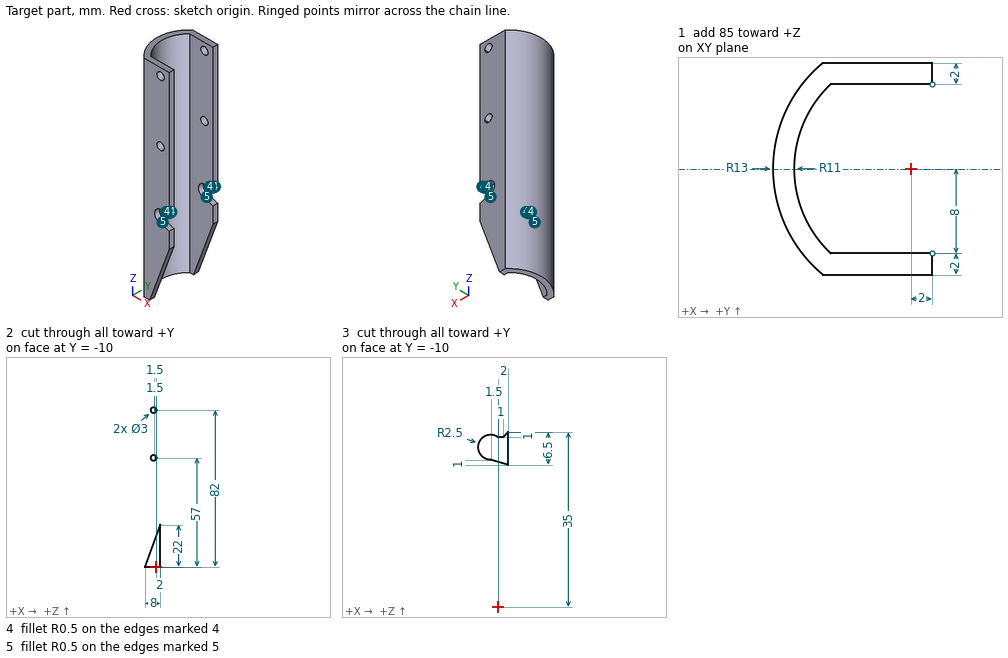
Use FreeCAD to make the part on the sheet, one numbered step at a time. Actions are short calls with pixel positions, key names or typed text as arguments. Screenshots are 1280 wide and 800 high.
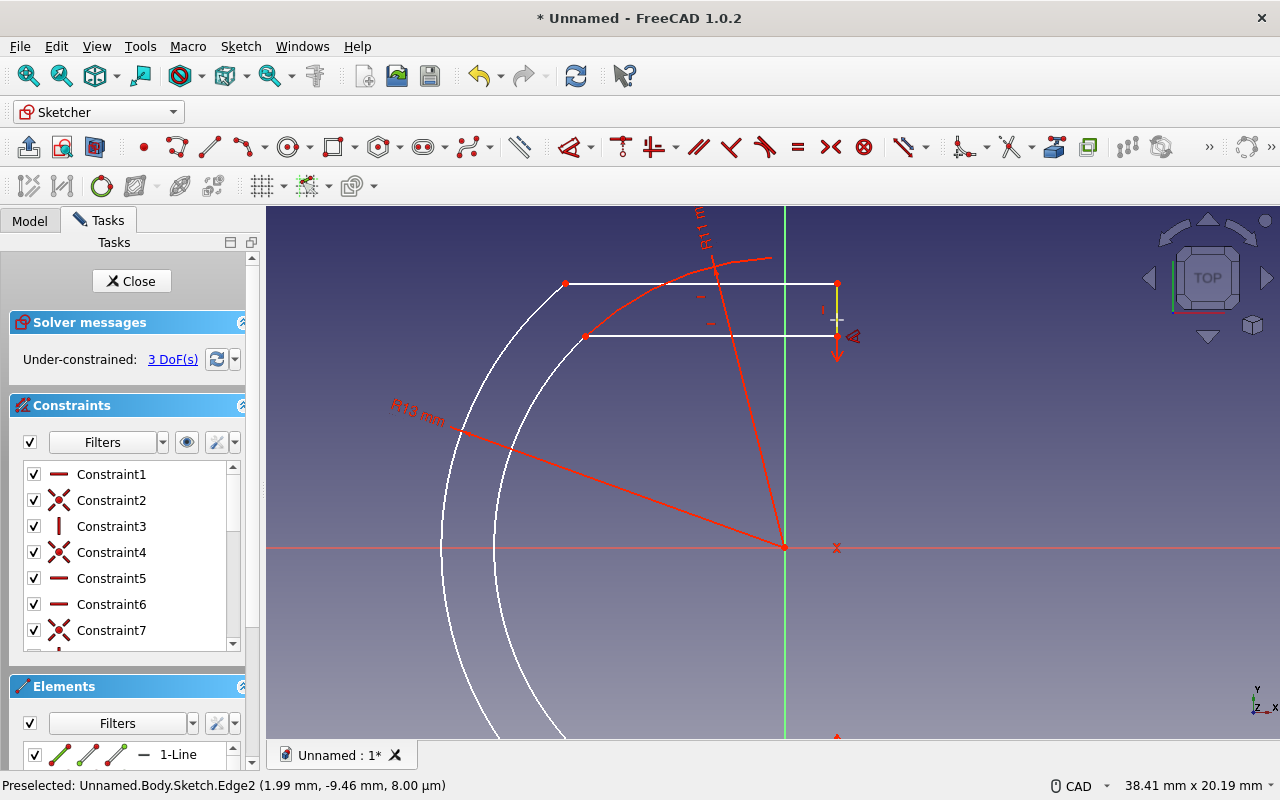
click(837, 320)
click(871, 310)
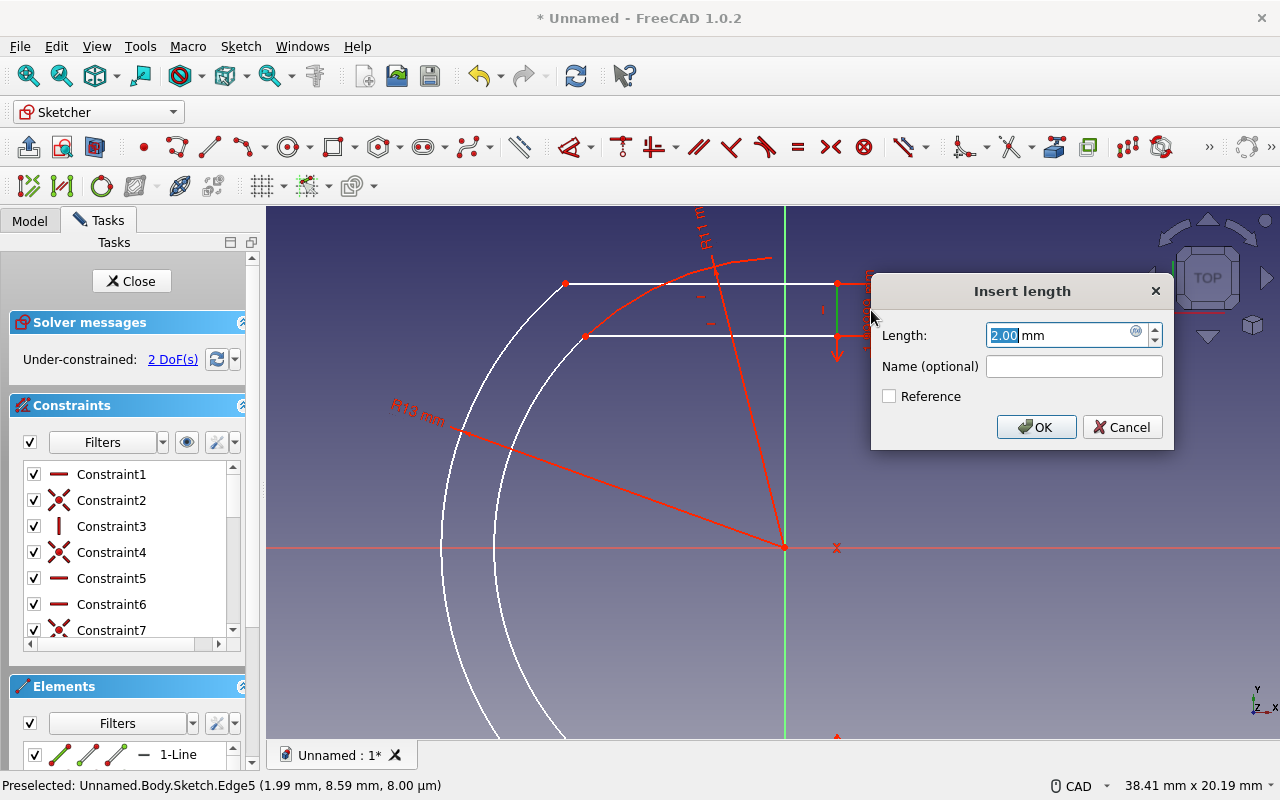
text(2)
key(Return)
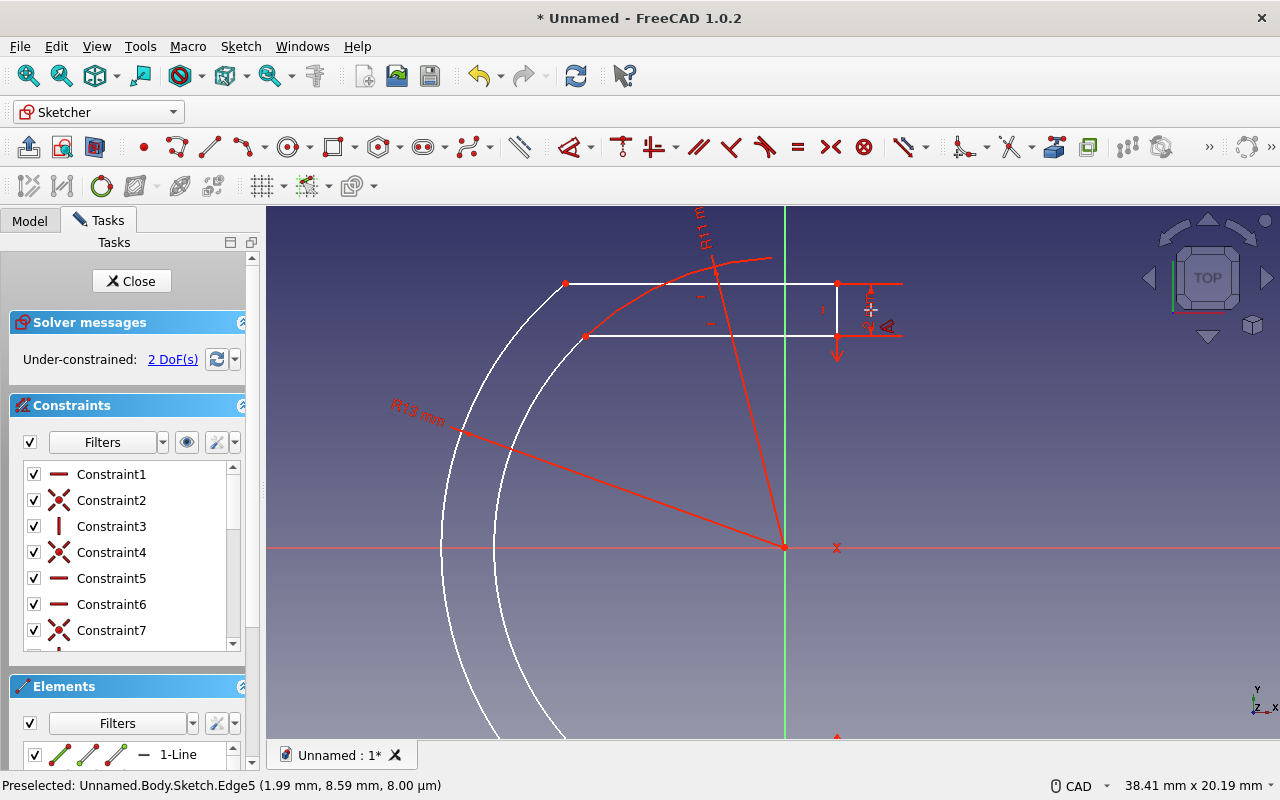
scroll(837, 319, down, 2)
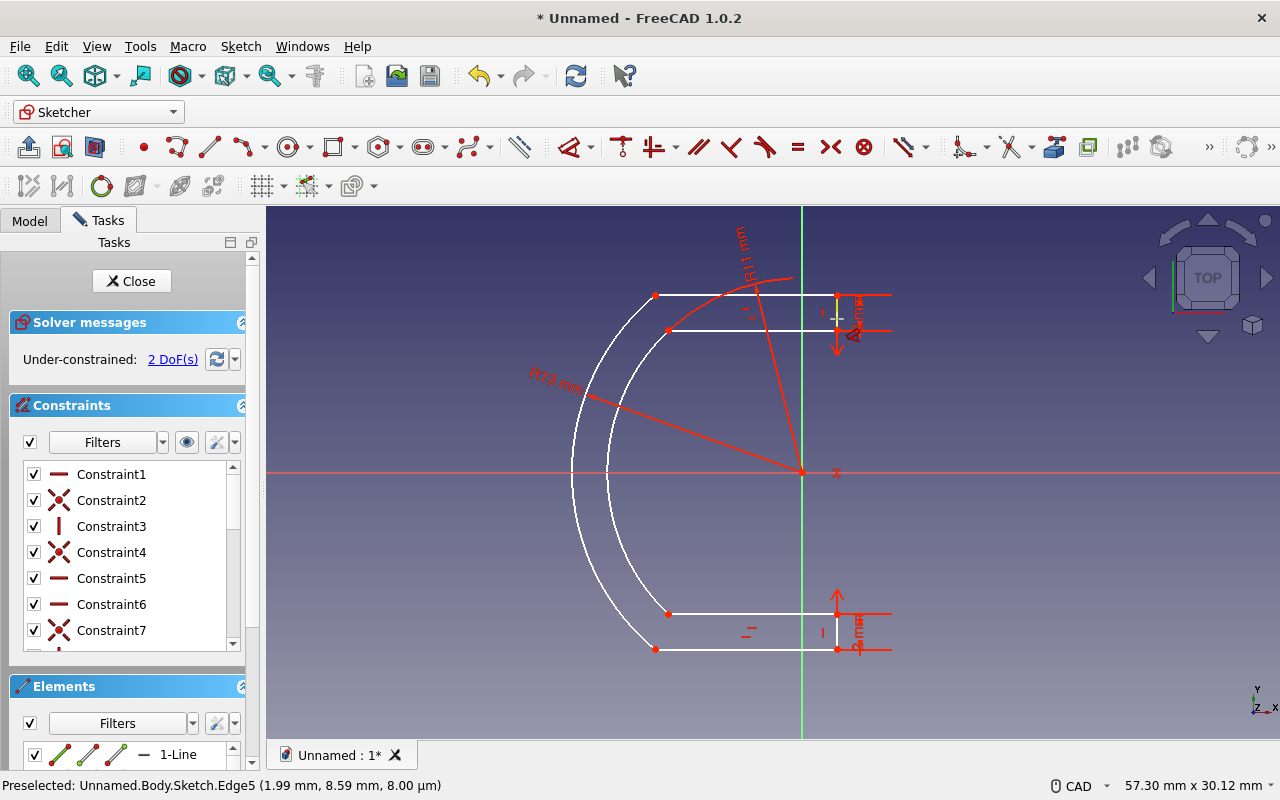
click(837, 650)
click(820, 684)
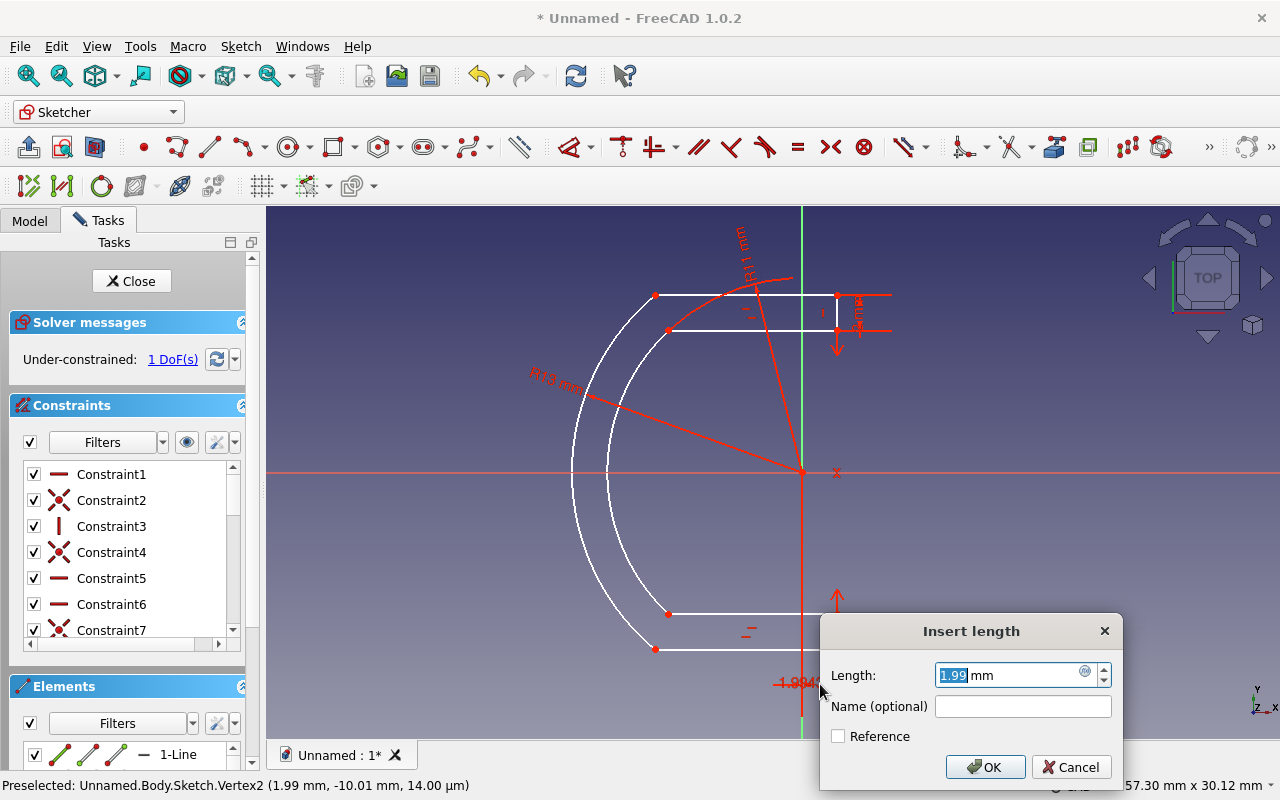
text(2)
key(Return)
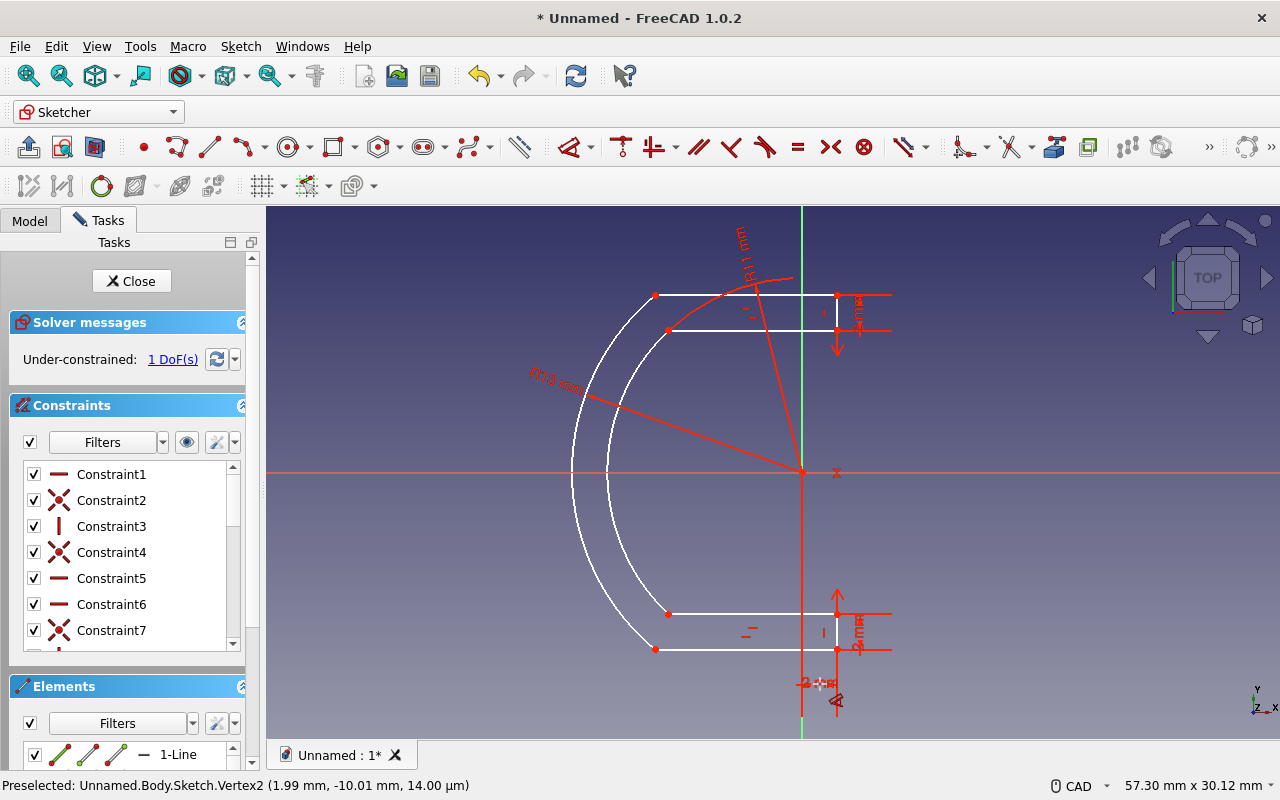
click(837, 614)
click(871, 543)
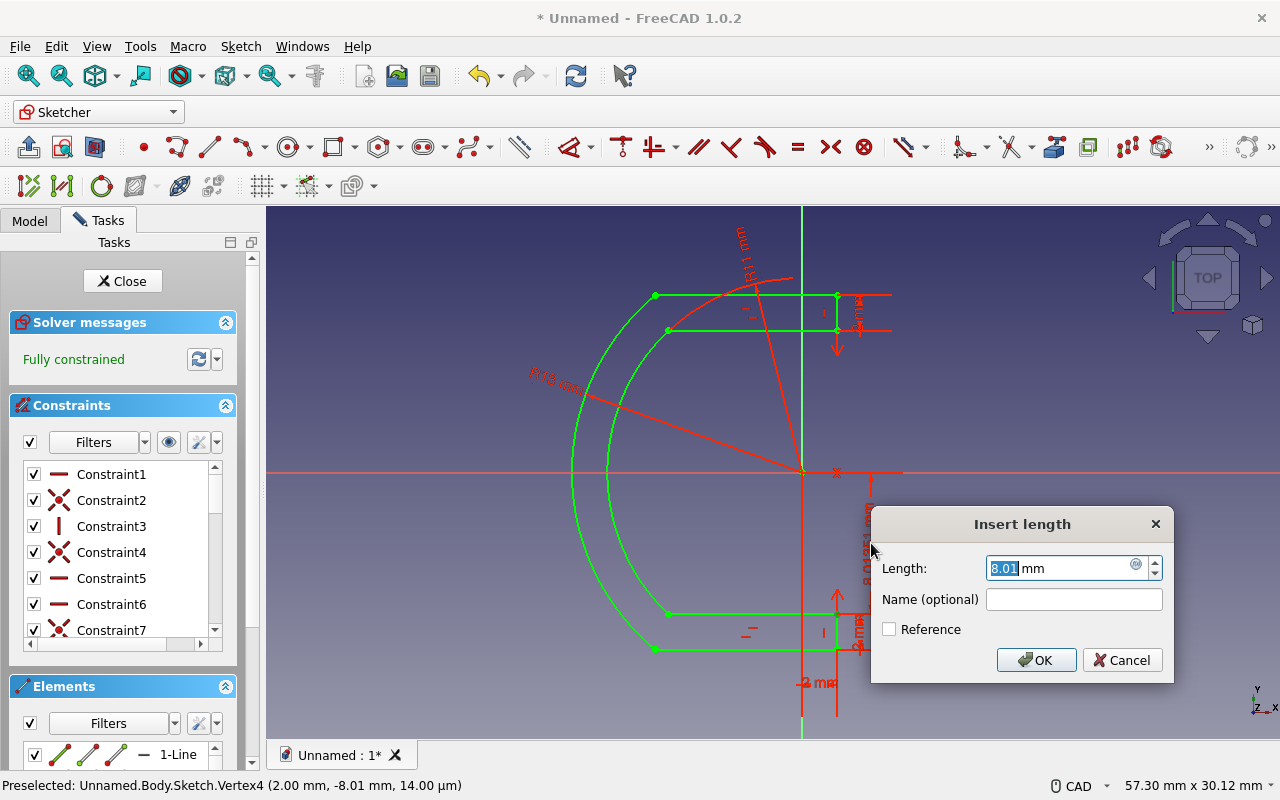
text(8)
key(Return)
key(Escape)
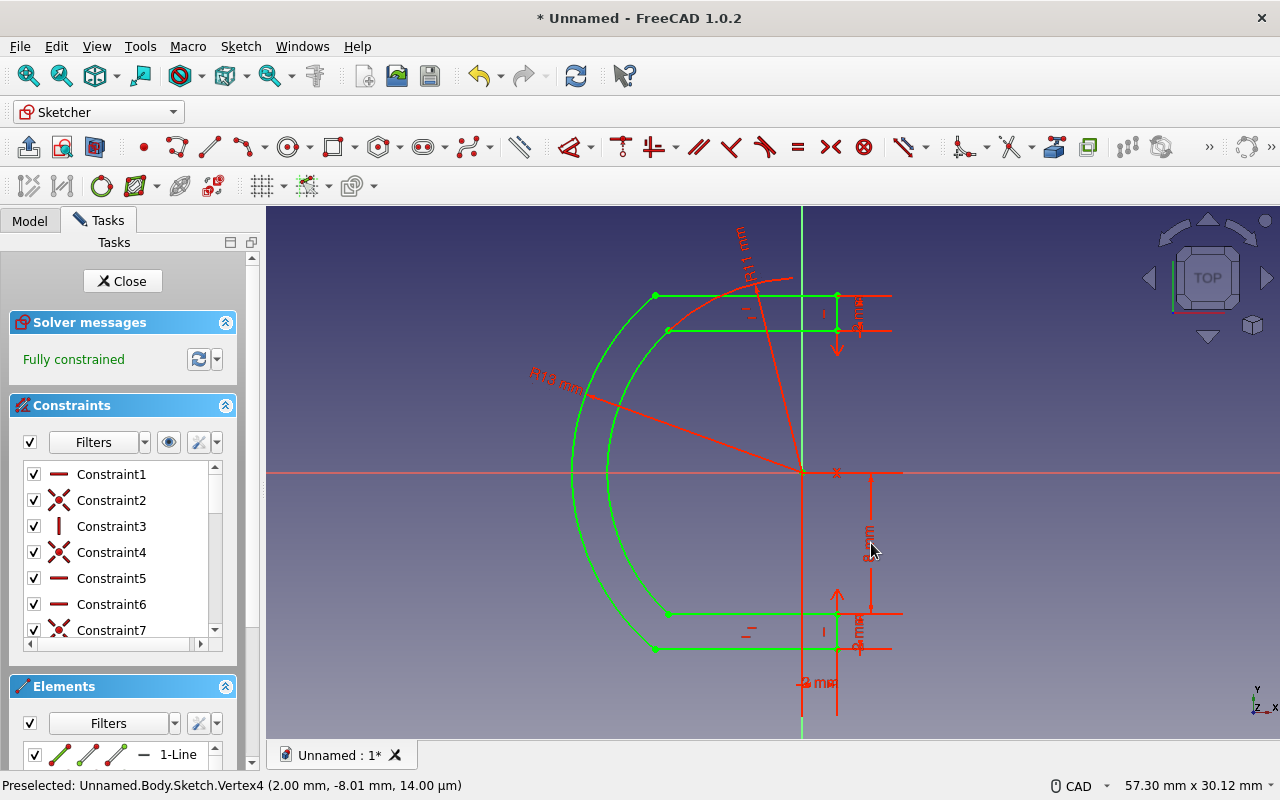
click(123, 281)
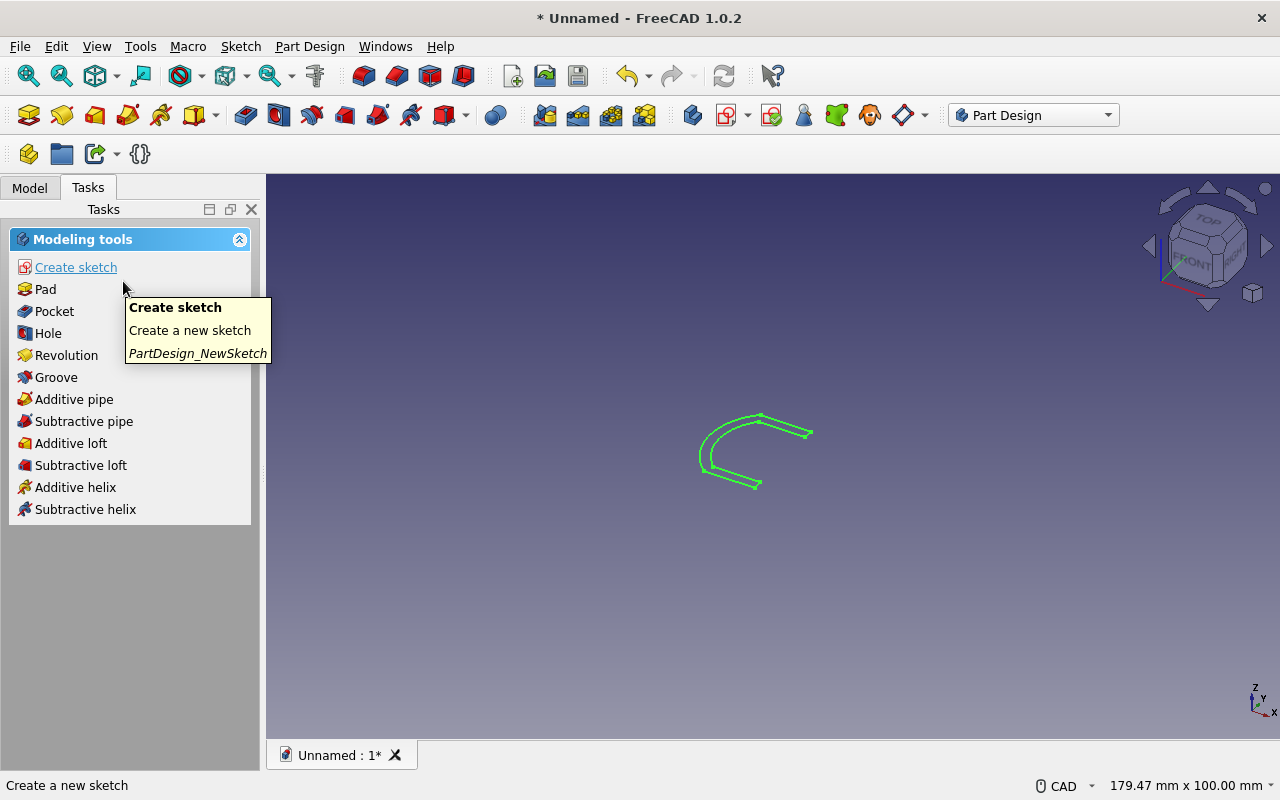
click(29, 116)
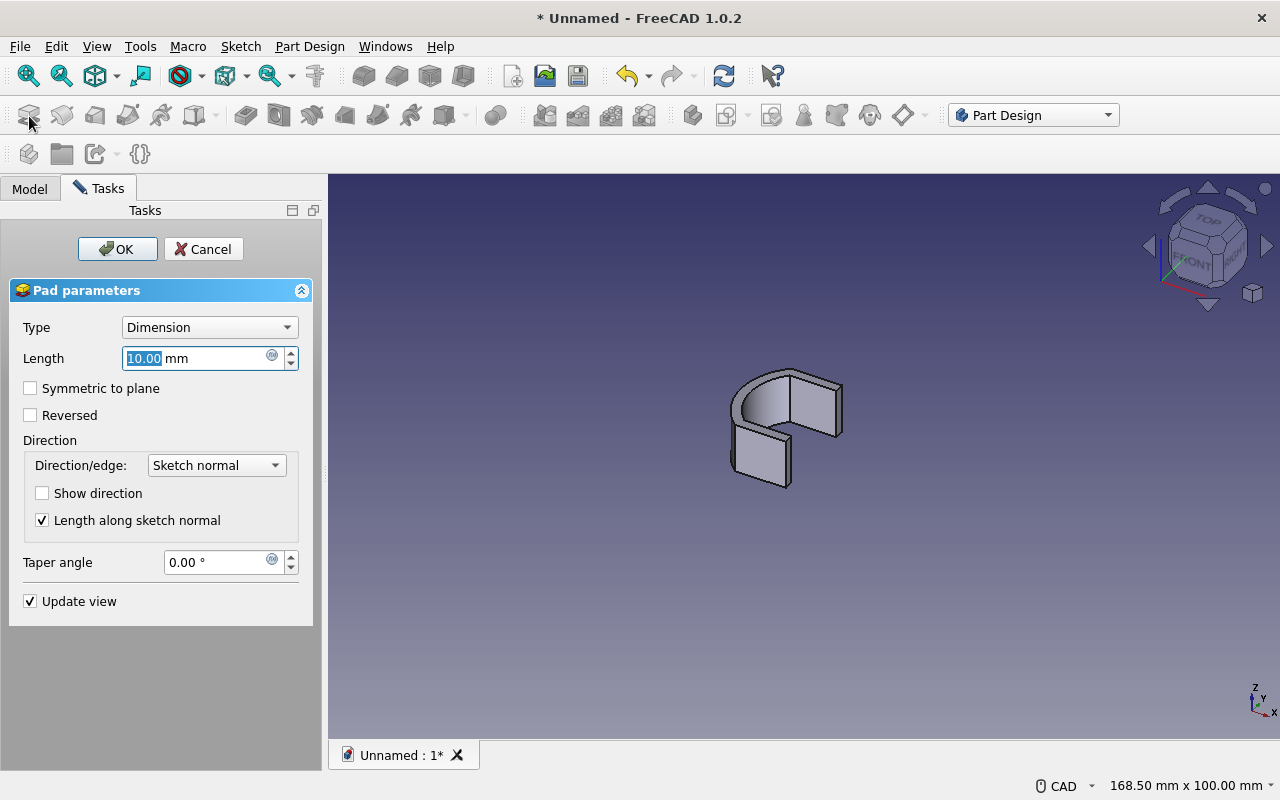
text(85)
key(Tab)